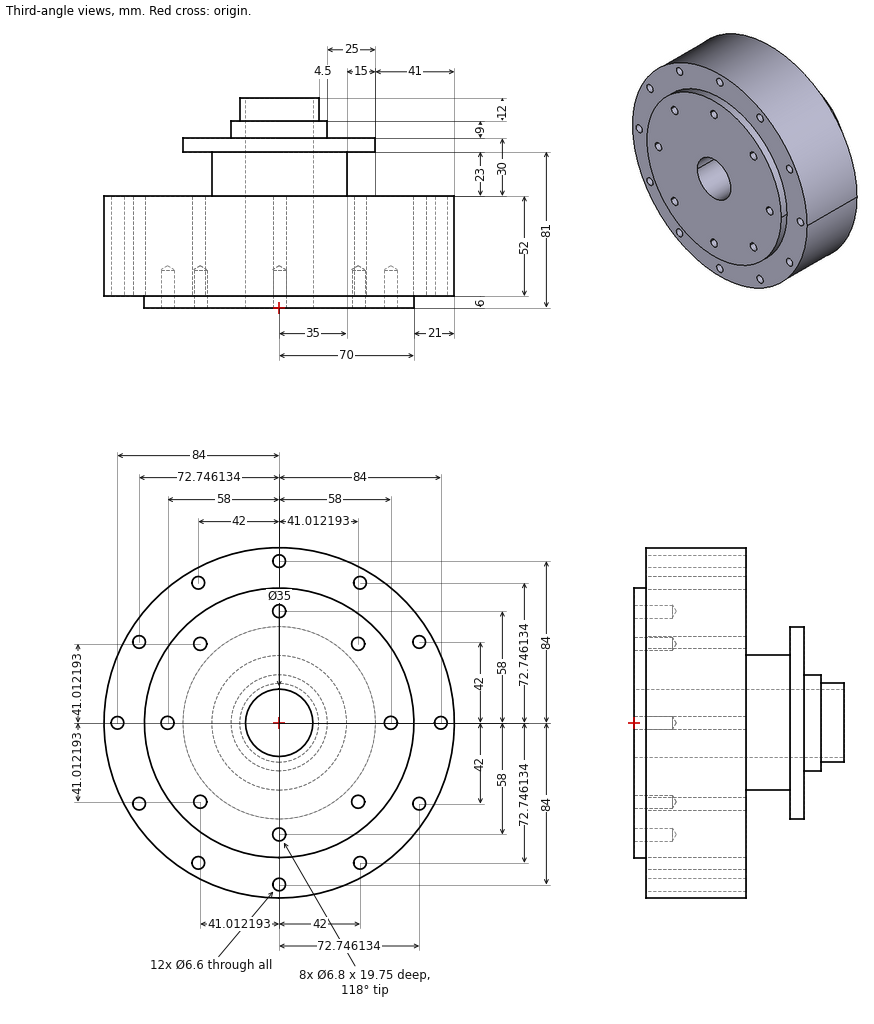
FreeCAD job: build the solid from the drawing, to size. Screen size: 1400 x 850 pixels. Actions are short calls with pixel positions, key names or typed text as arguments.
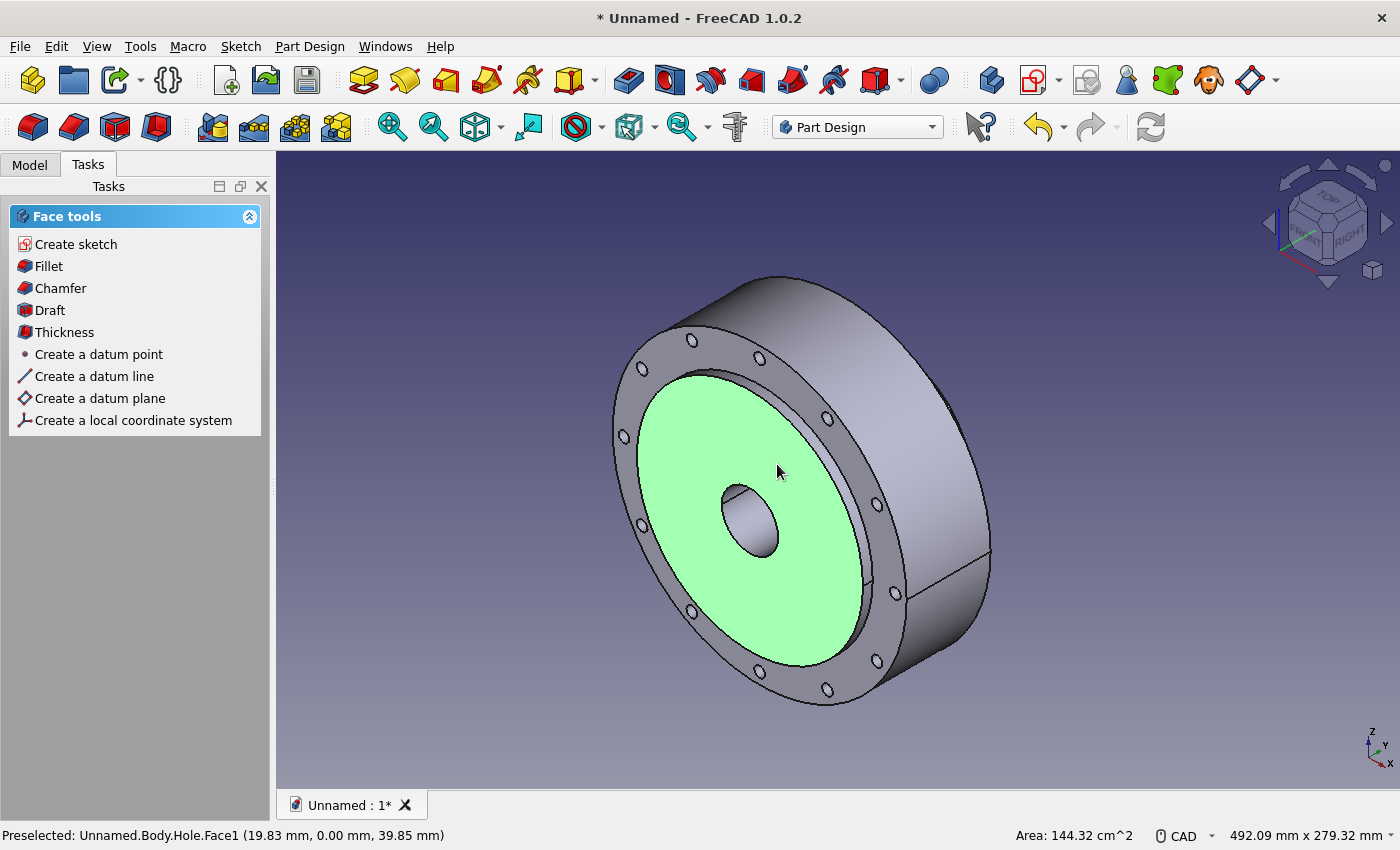
click(1032, 80)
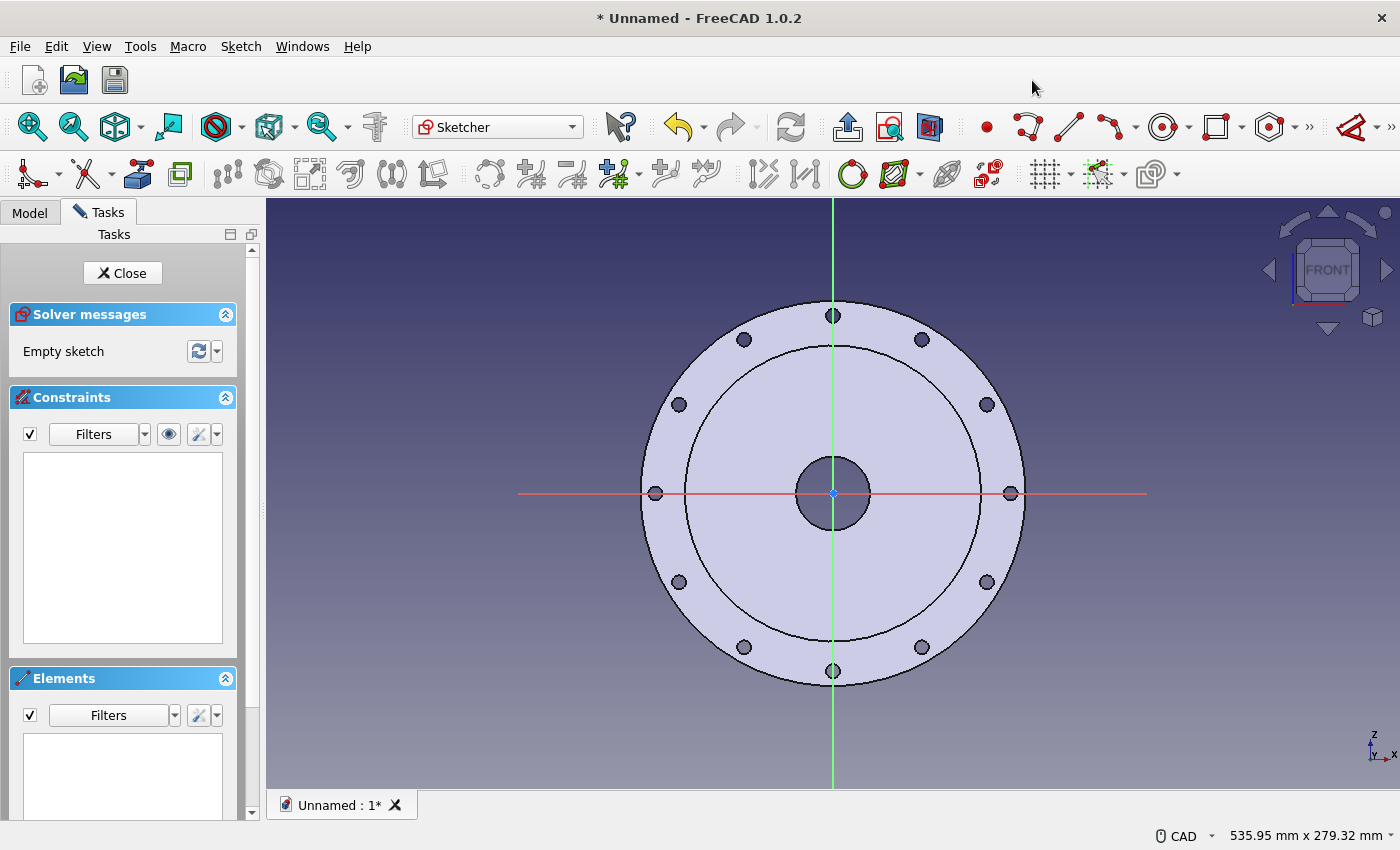
scroll(972, 494, up, 2)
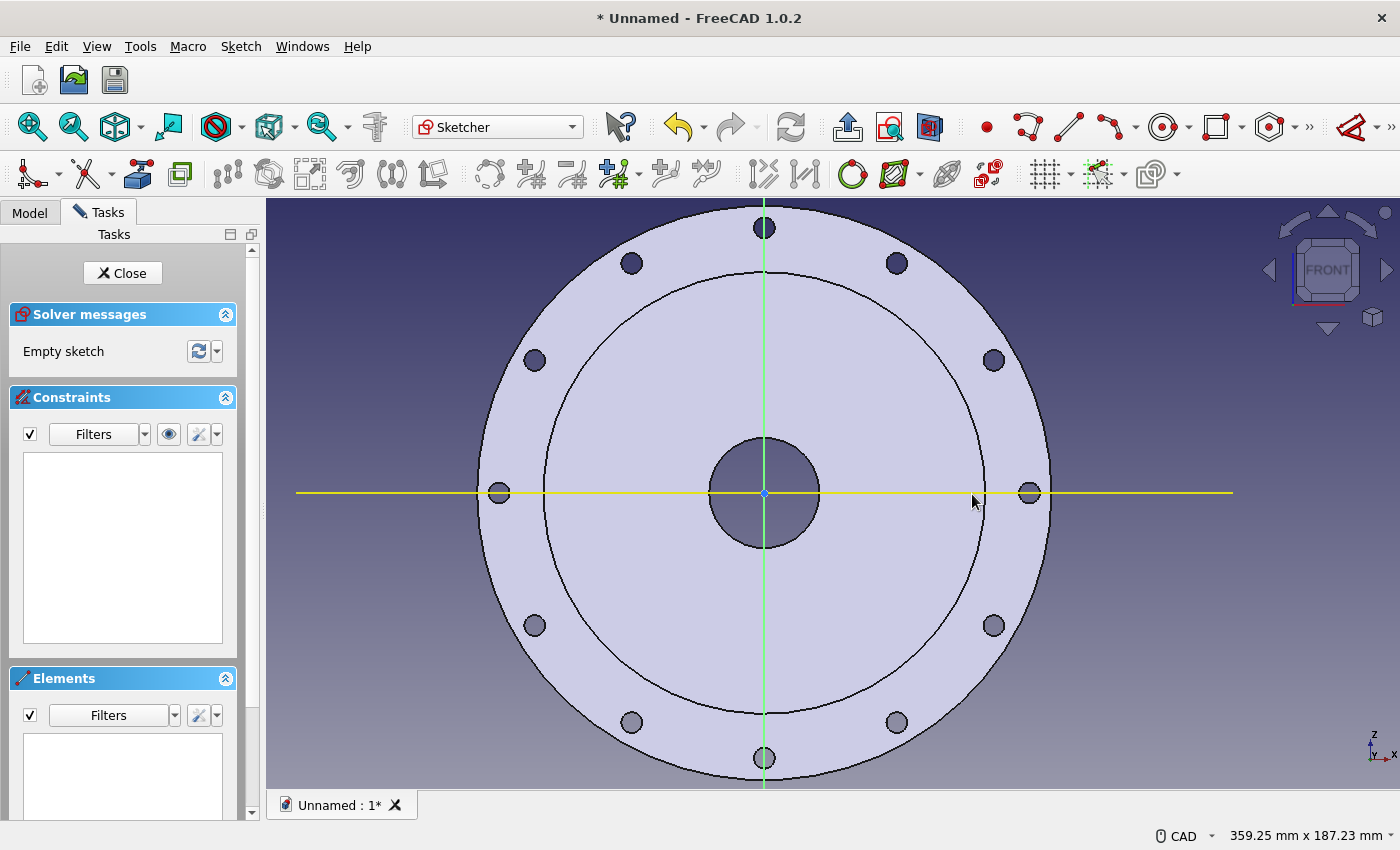
key(g)
key(c)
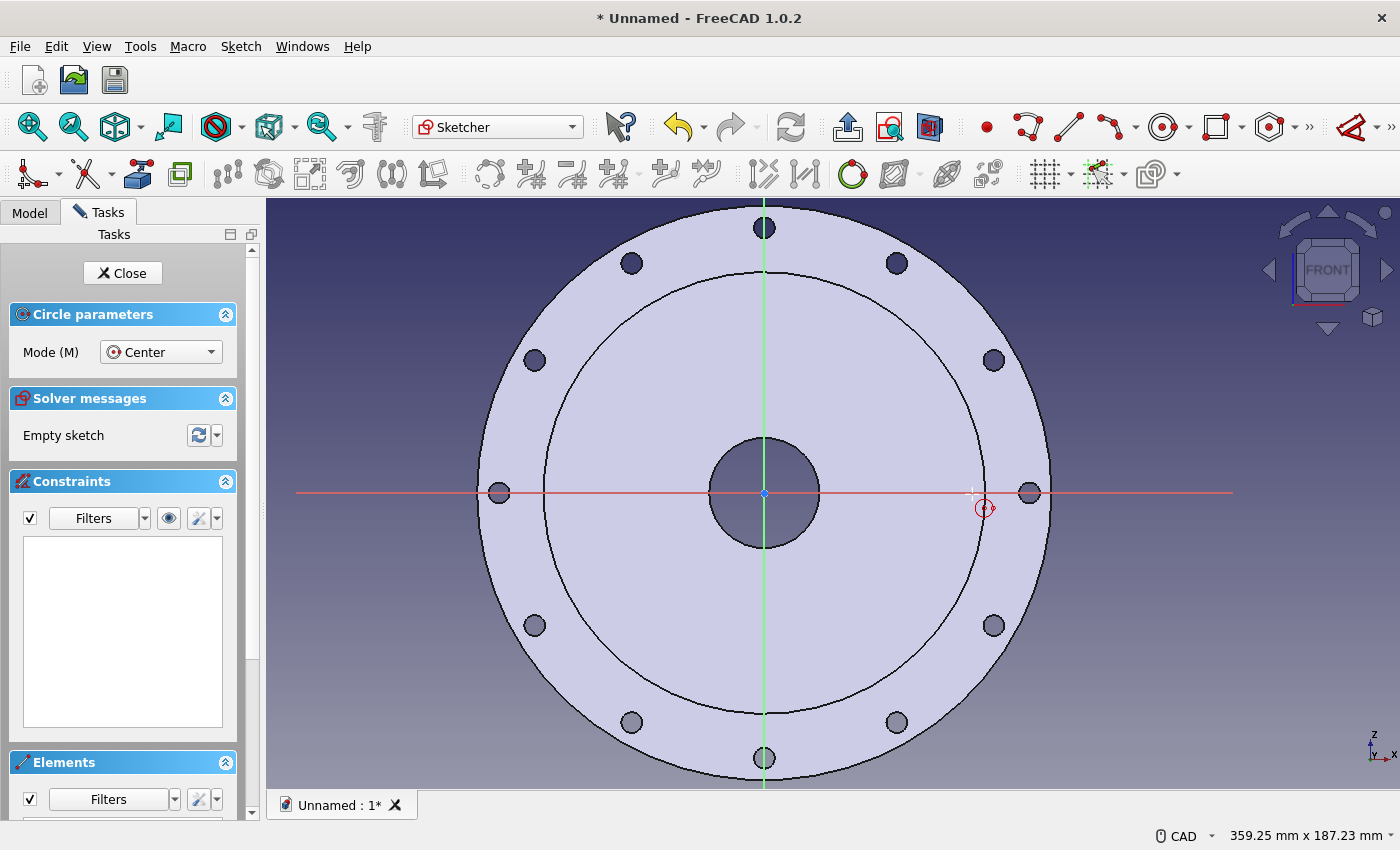
scroll(764, 676, up, 4)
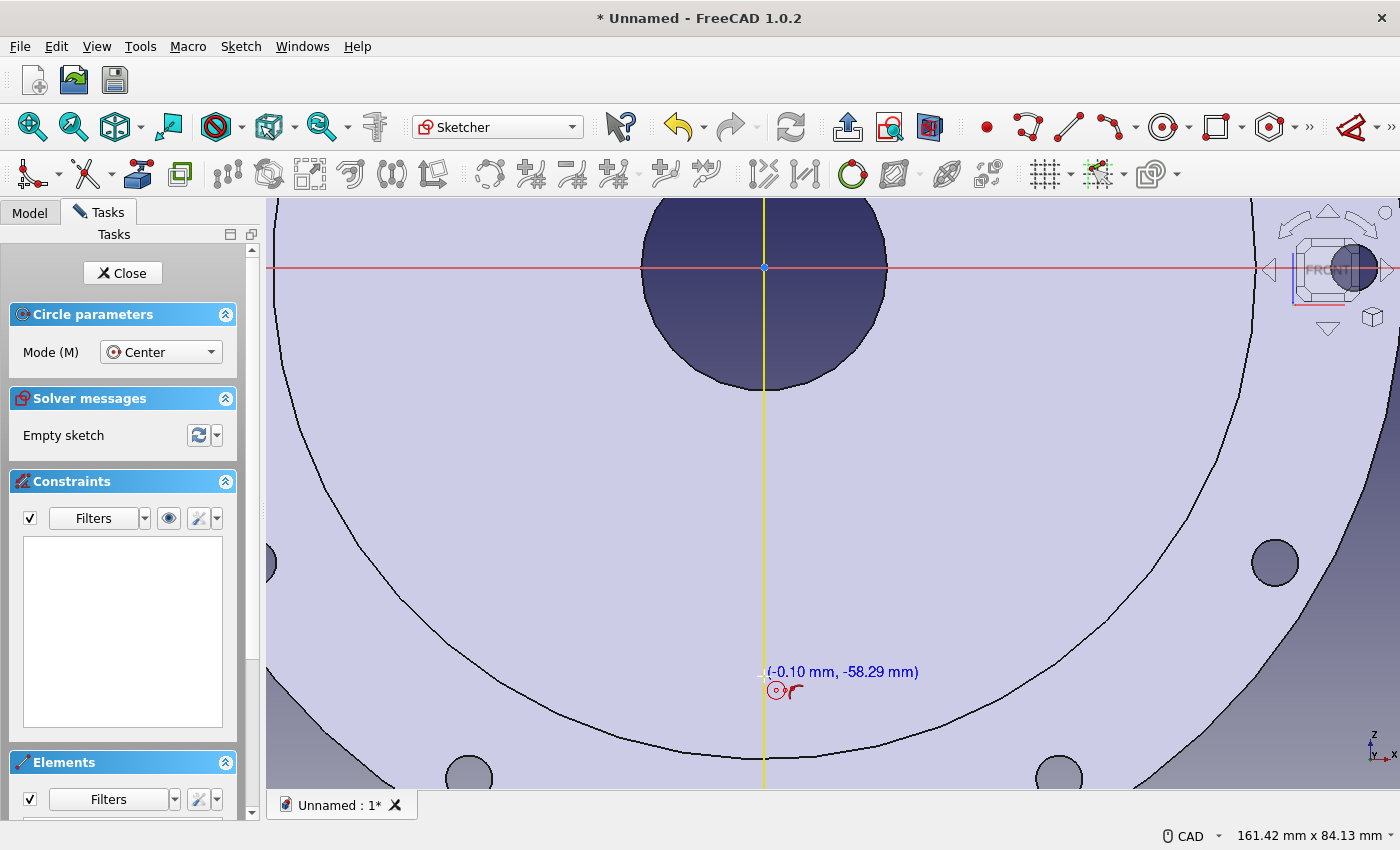
click(764, 675)
click(781, 658)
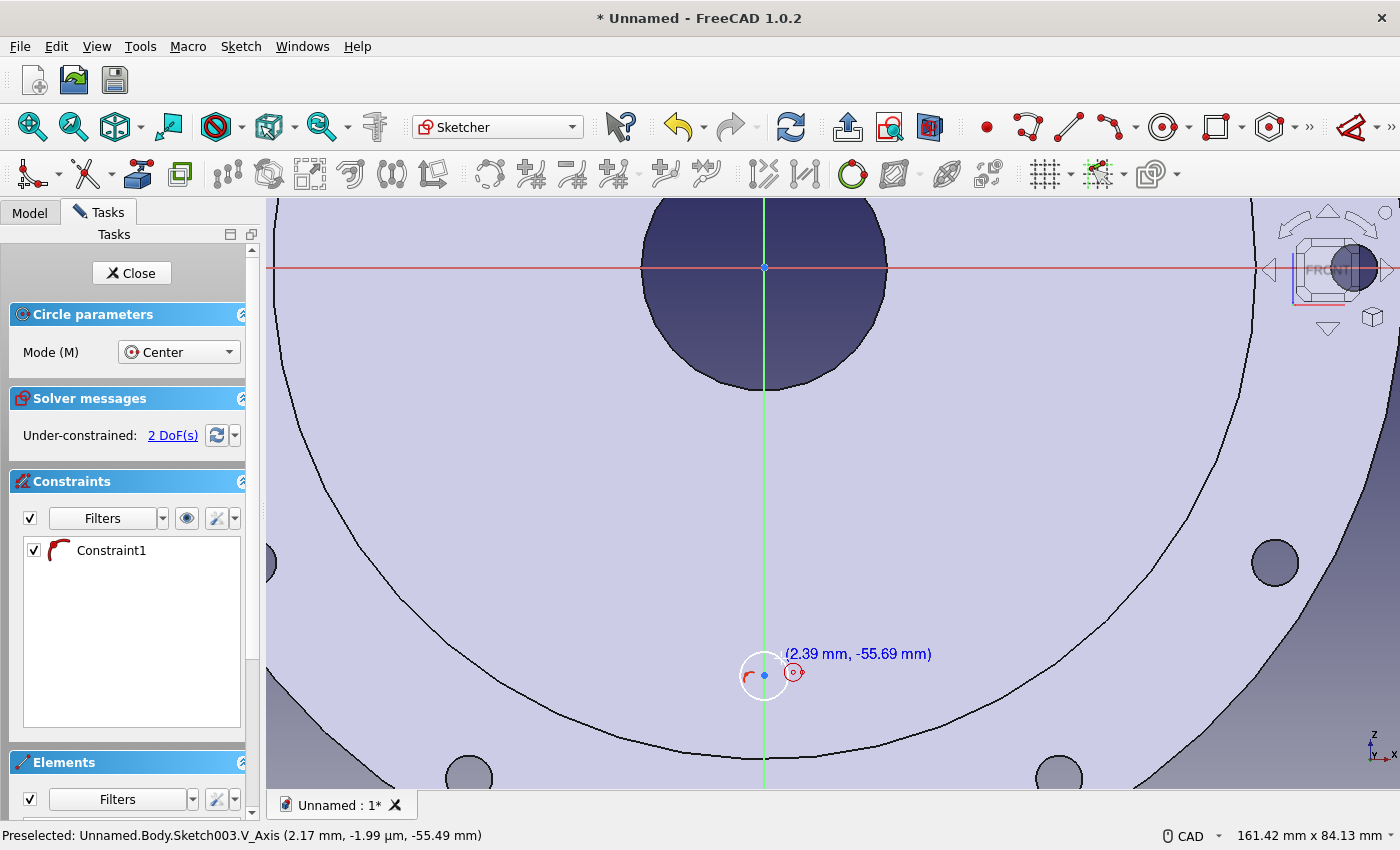
click(476, 556)
click(493, 539)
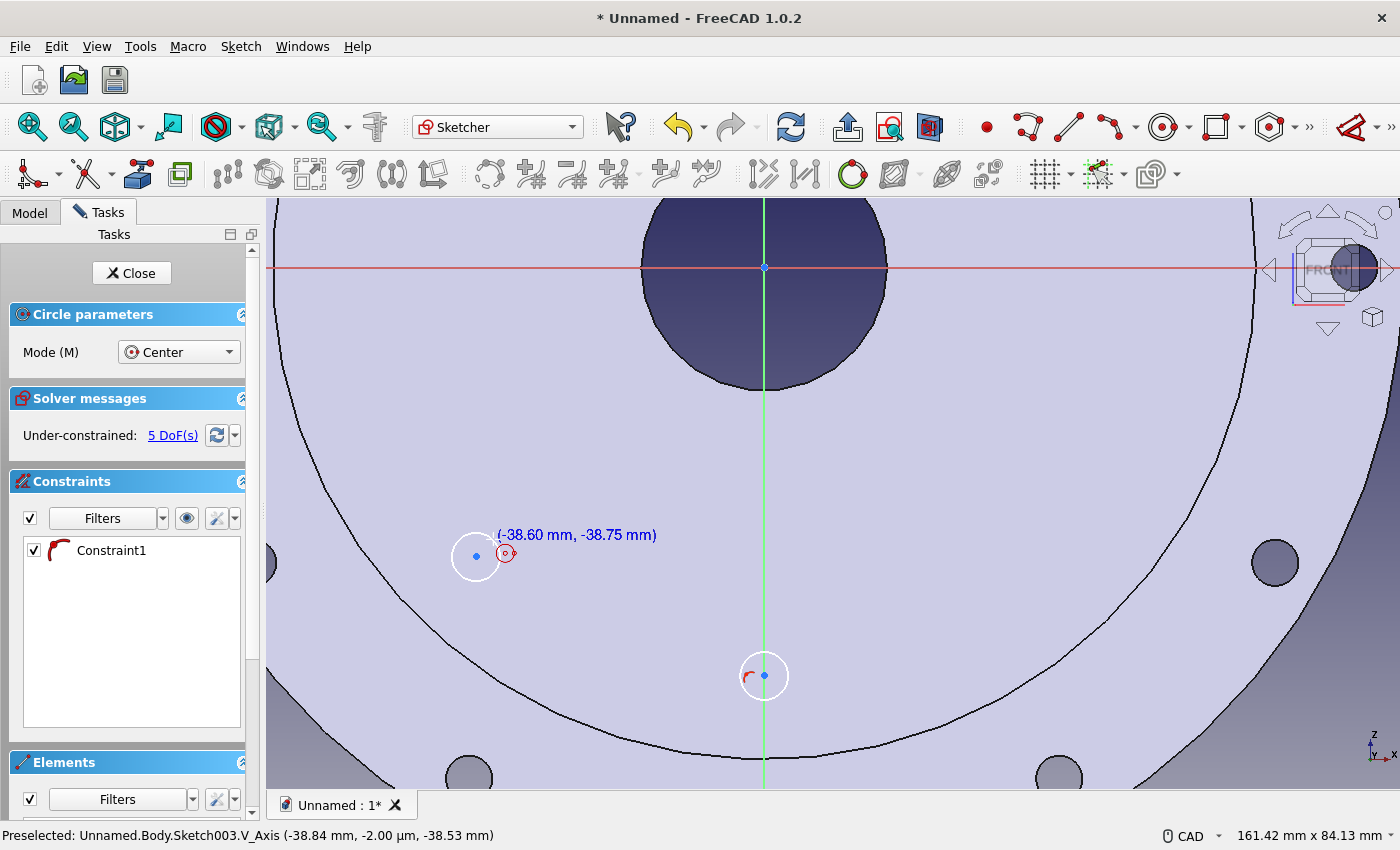
click(357, 268)
click(374, 251)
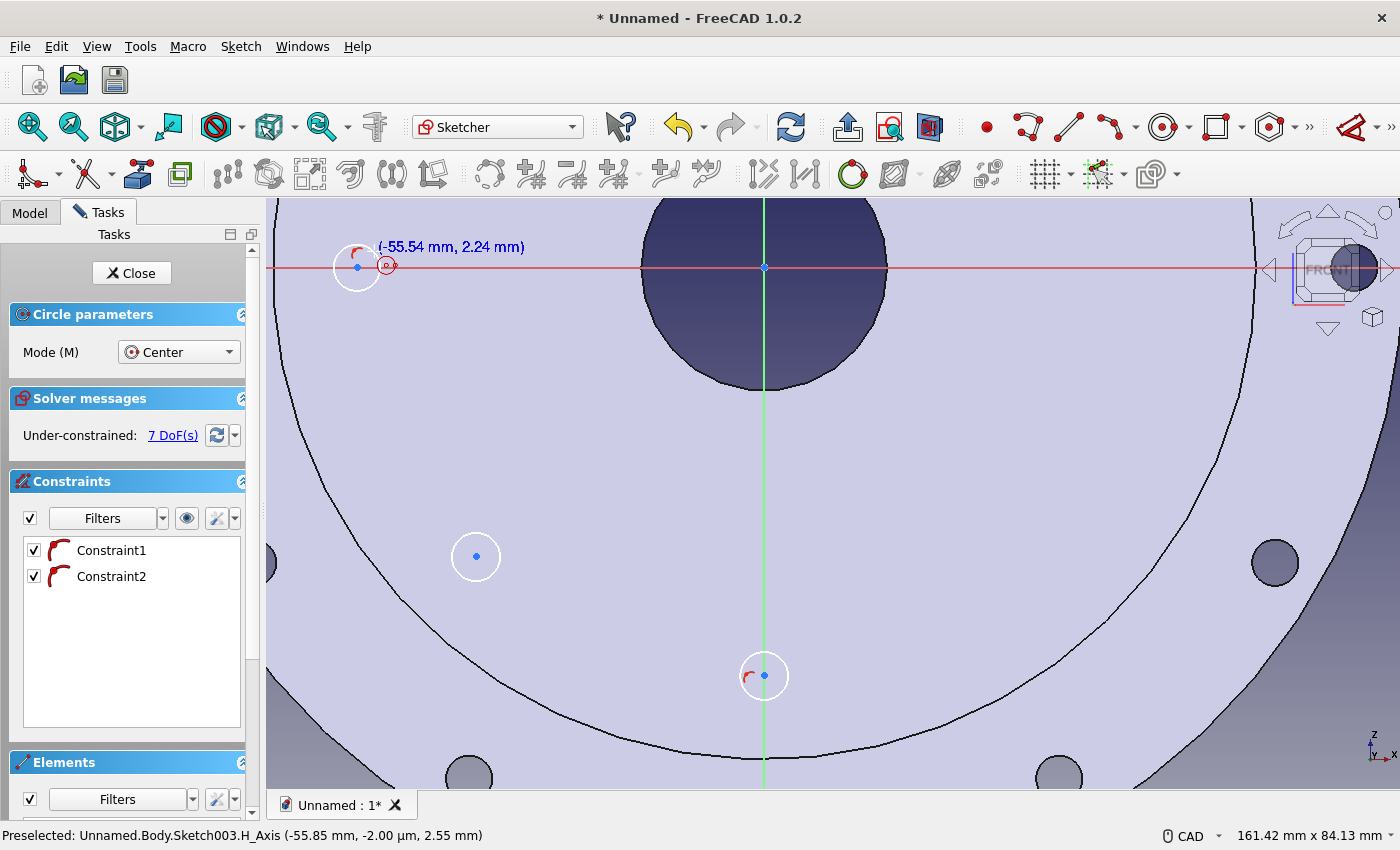
scroll(765, 678, down, 4)